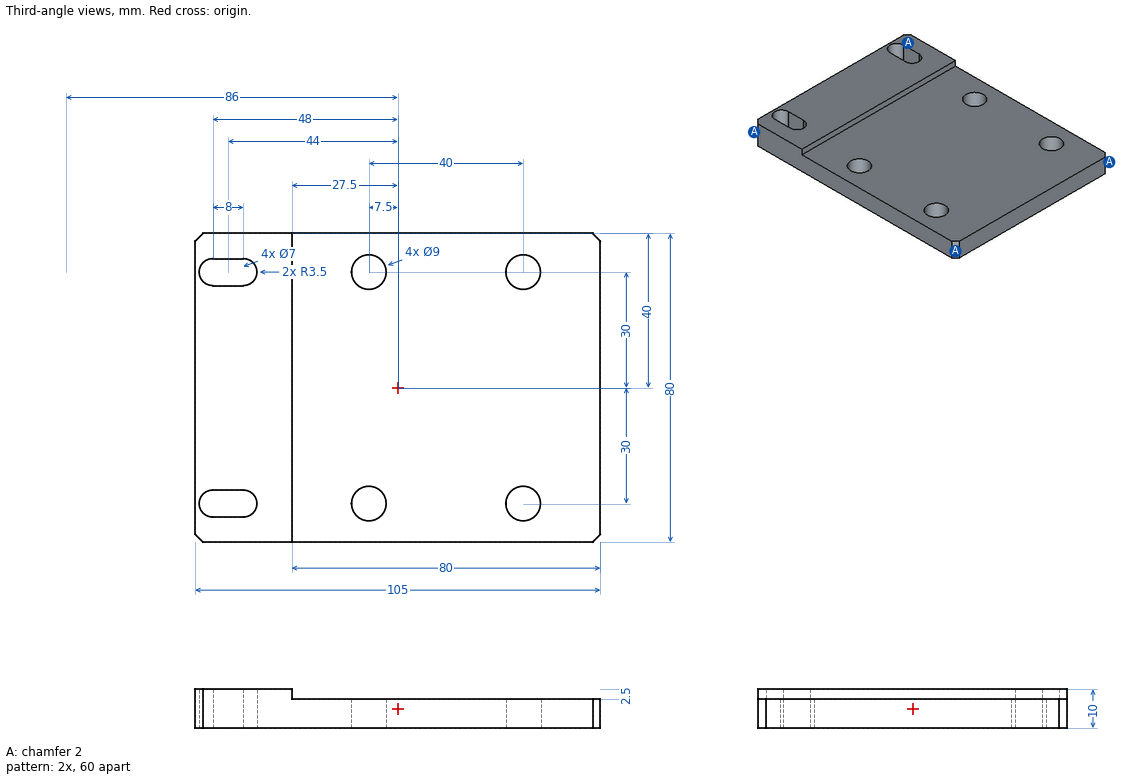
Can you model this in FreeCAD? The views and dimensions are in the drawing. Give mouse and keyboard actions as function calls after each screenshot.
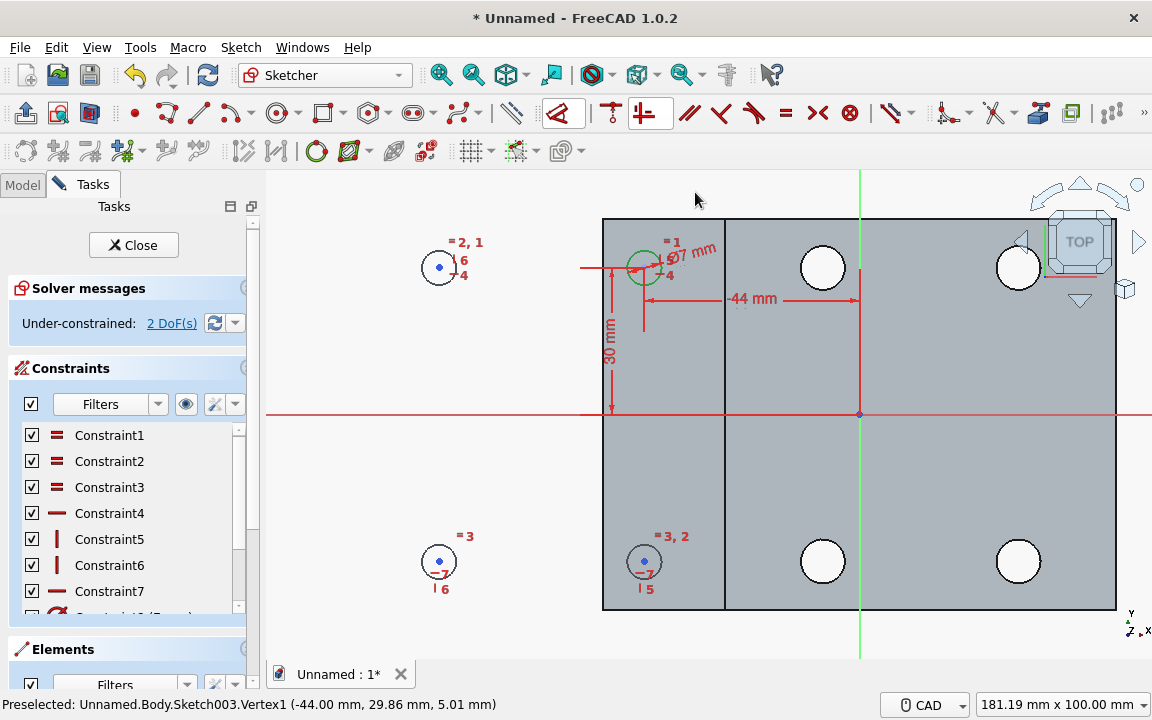
click(439, 268)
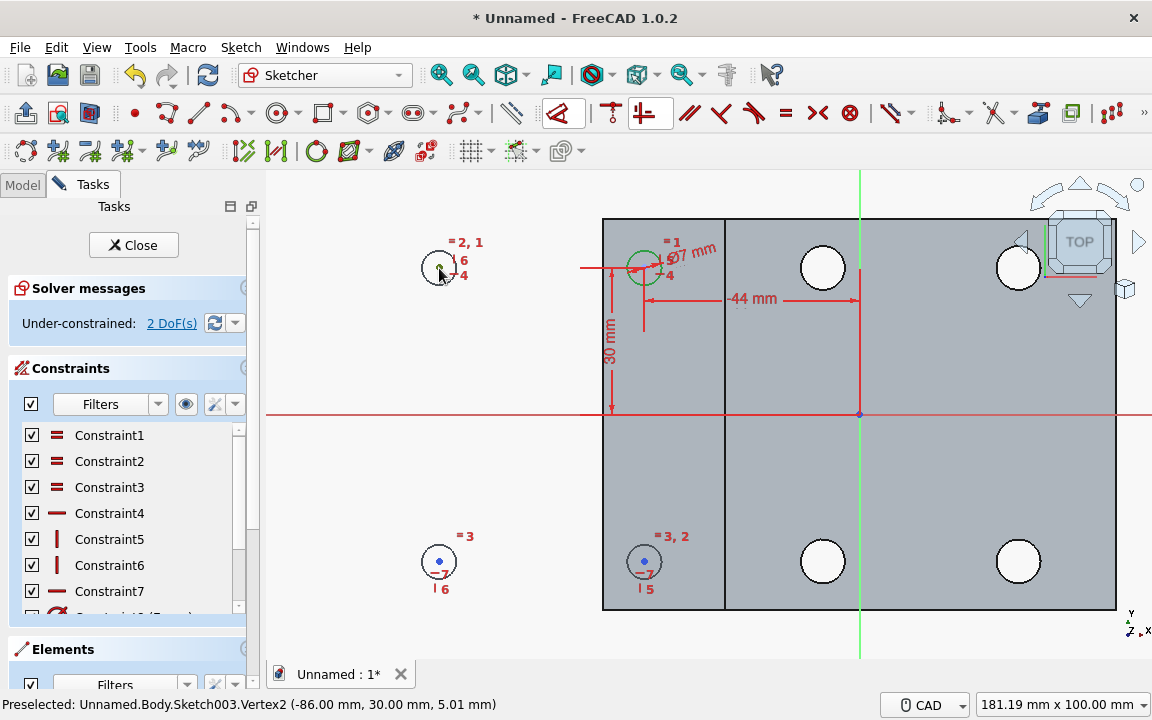
key(l)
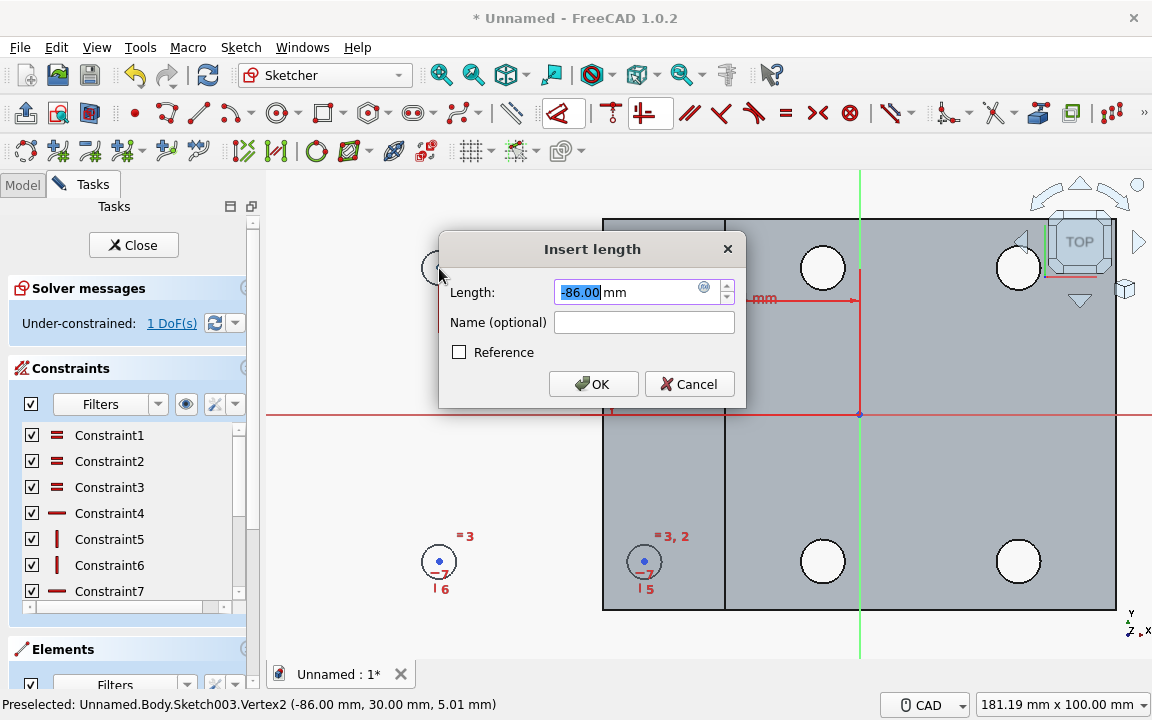
text(-86)
key(Return)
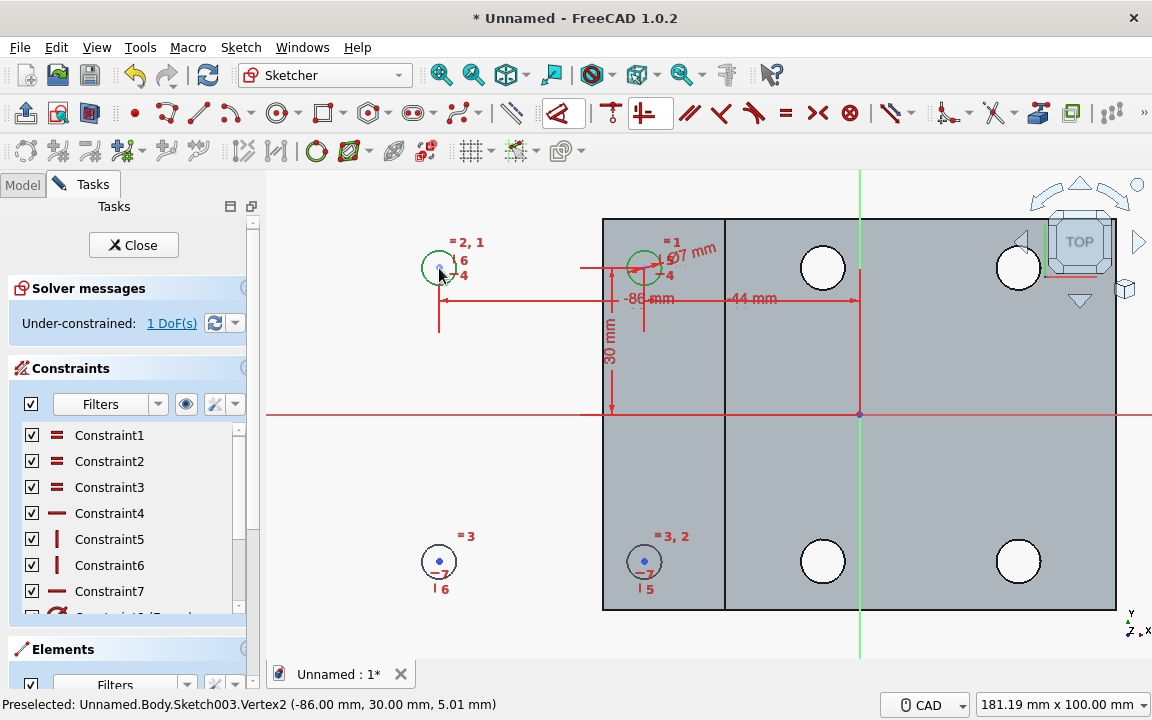
click(644, 562)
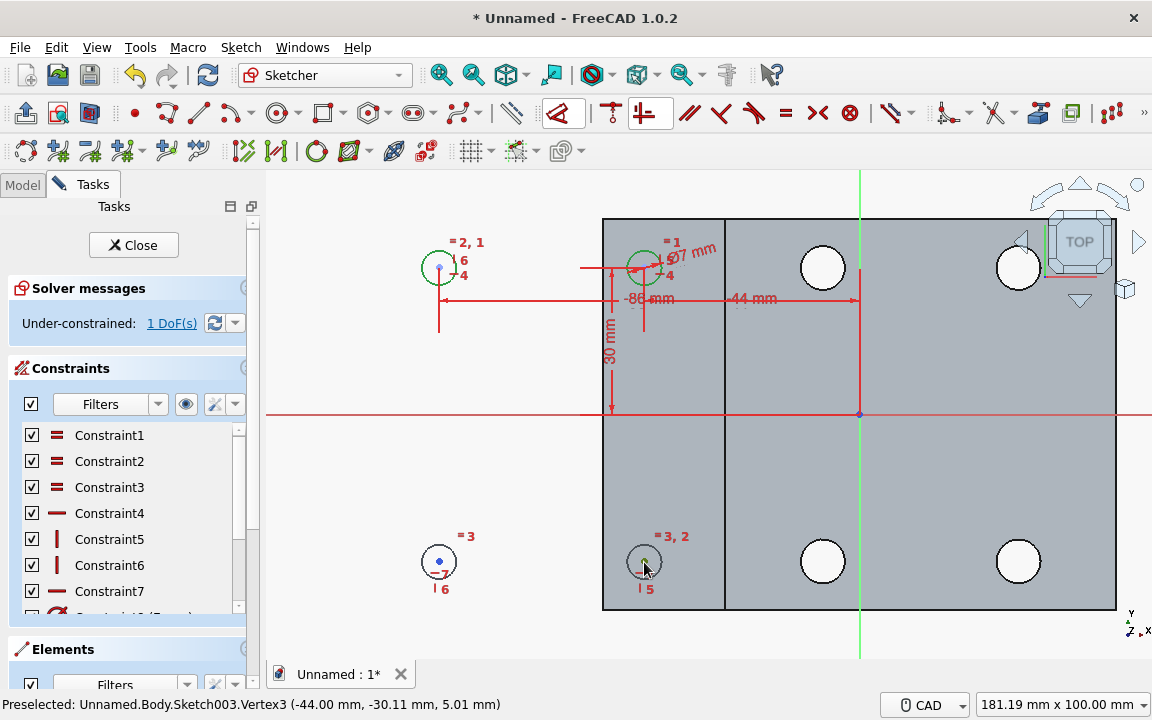
key(i)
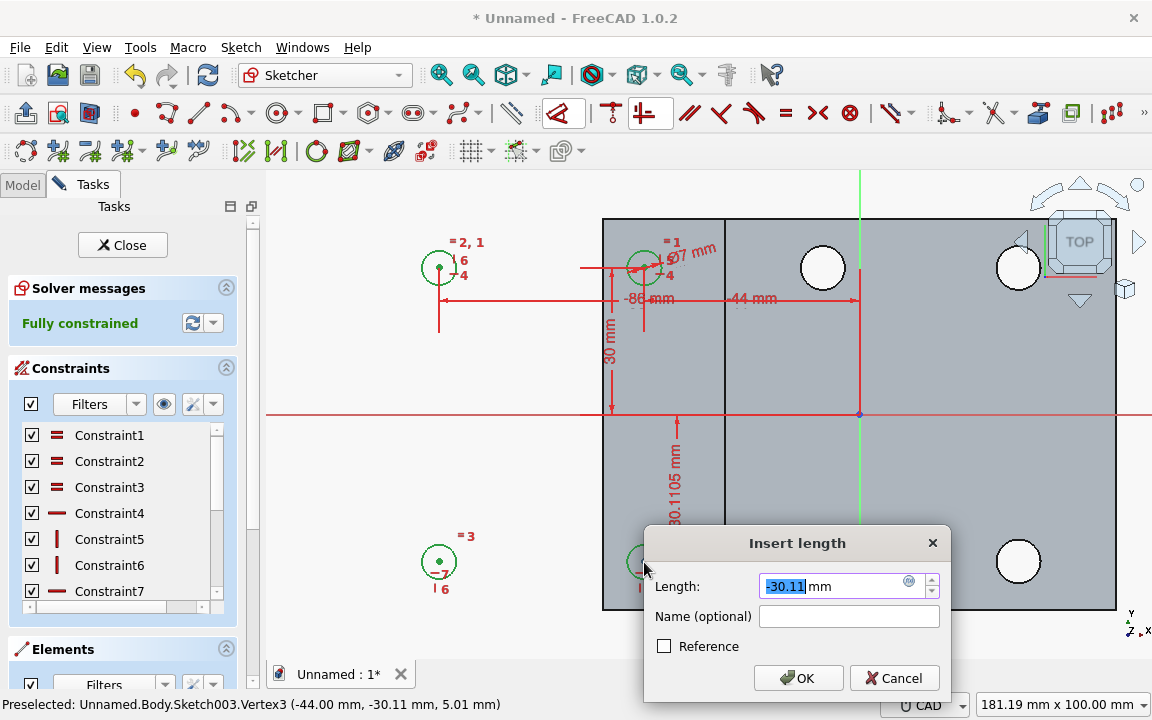
text(-30)
key(Return)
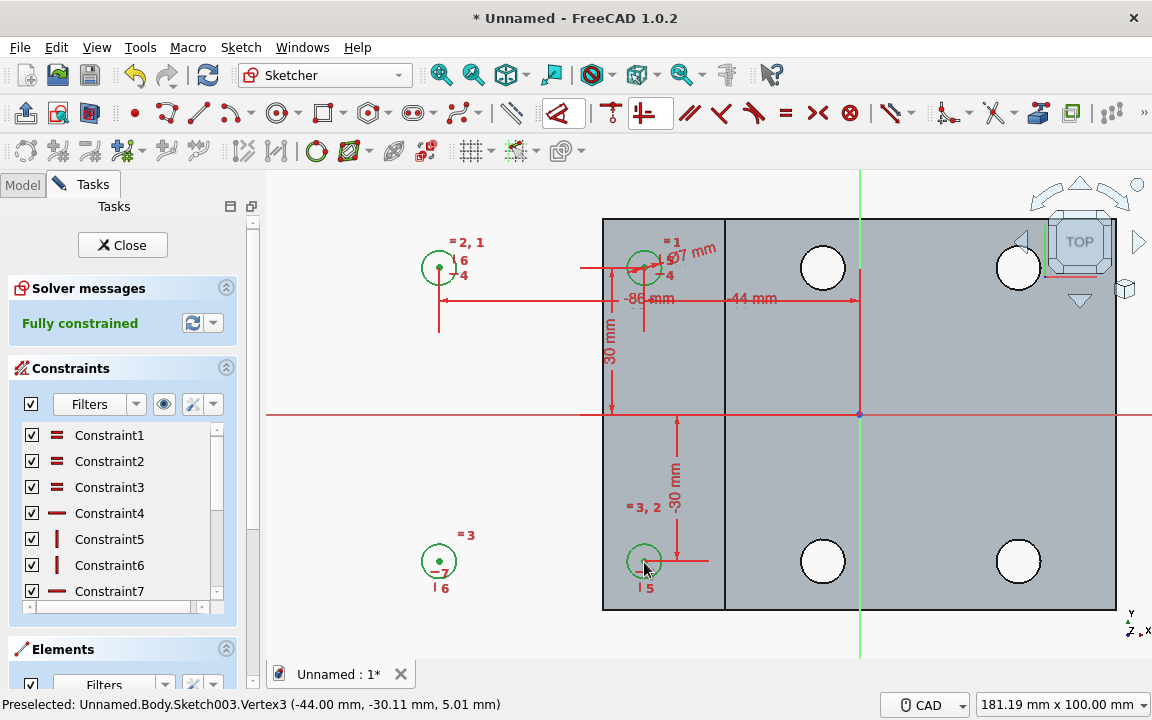
click(123, 245)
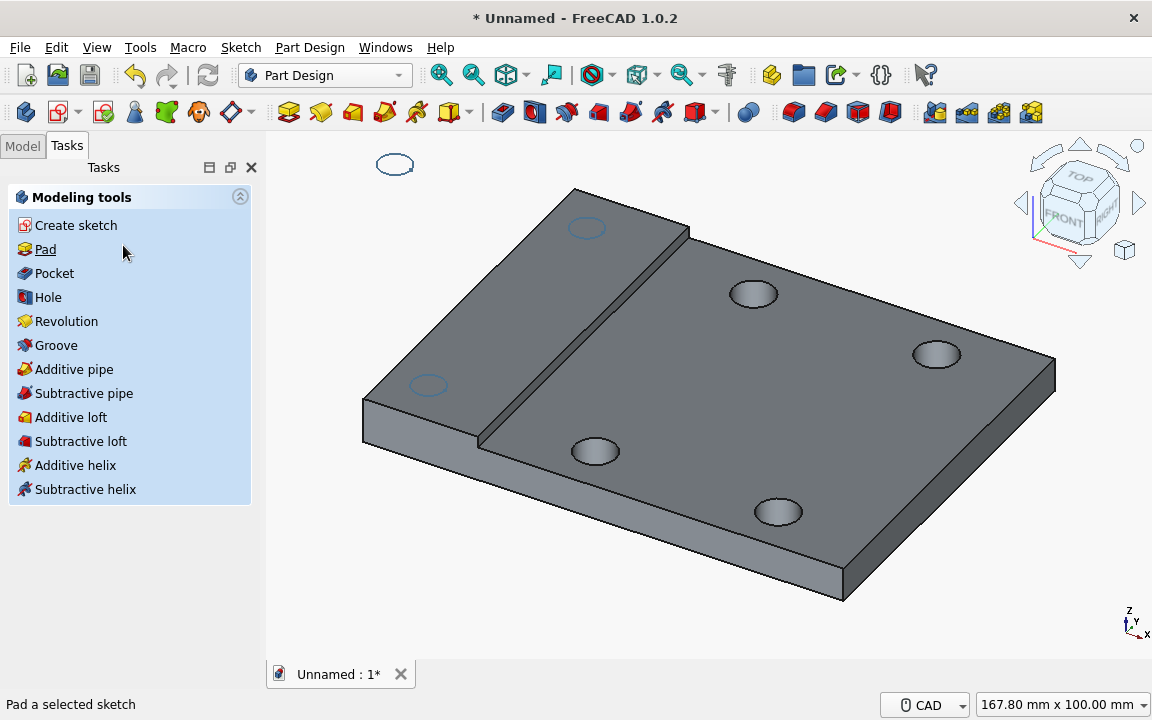
click(504, 112)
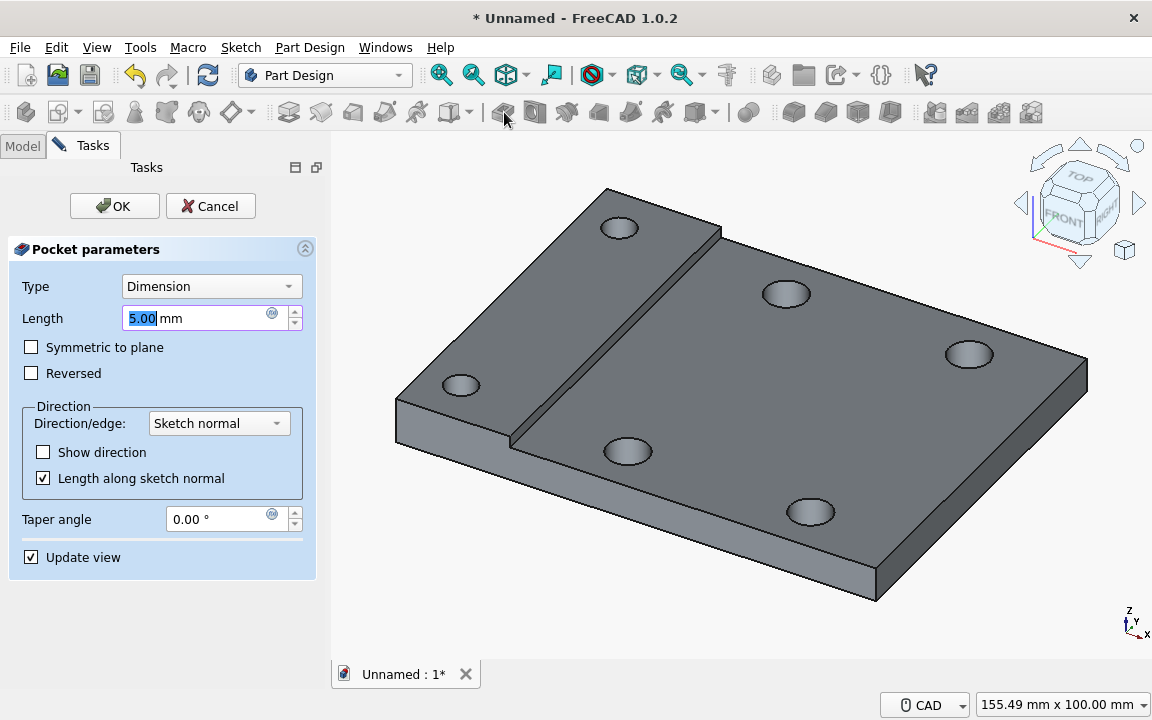
click(212, 286)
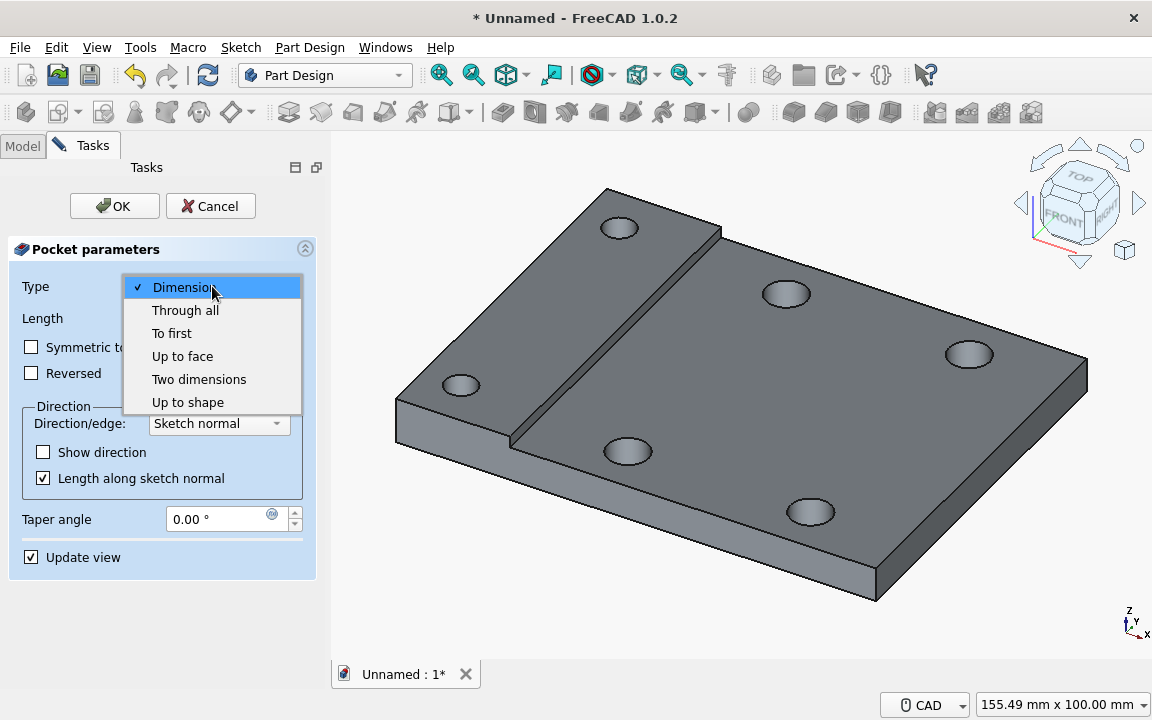
click(212, 310)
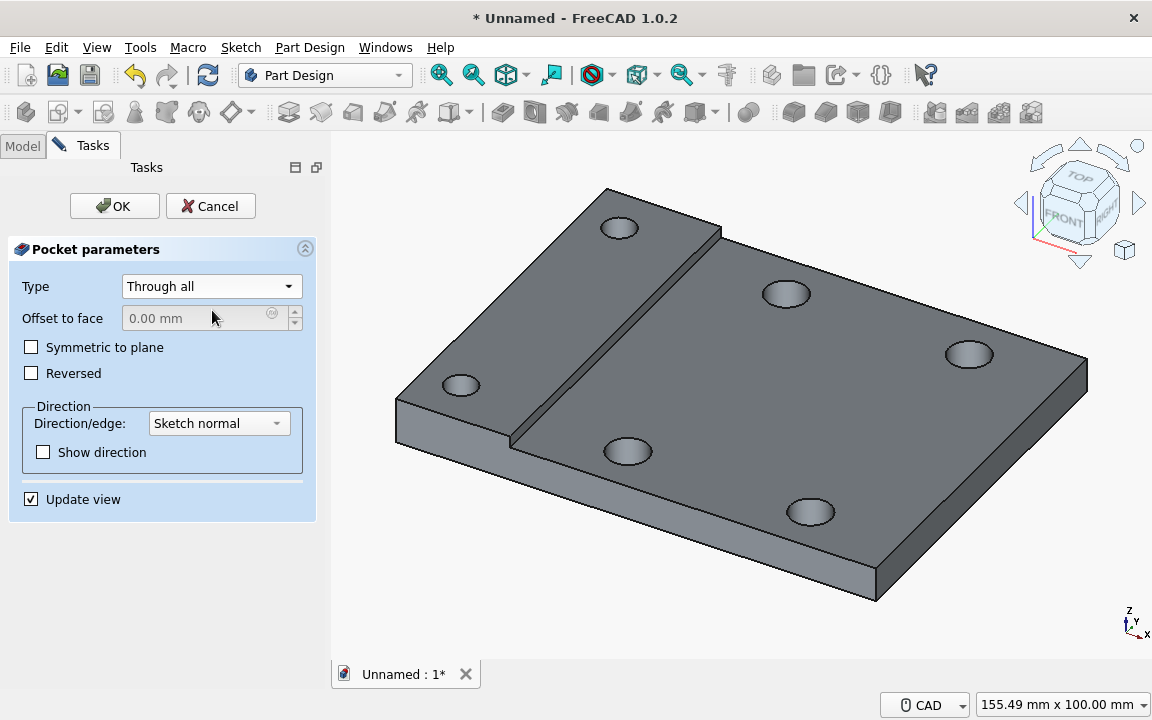
click(115, 206)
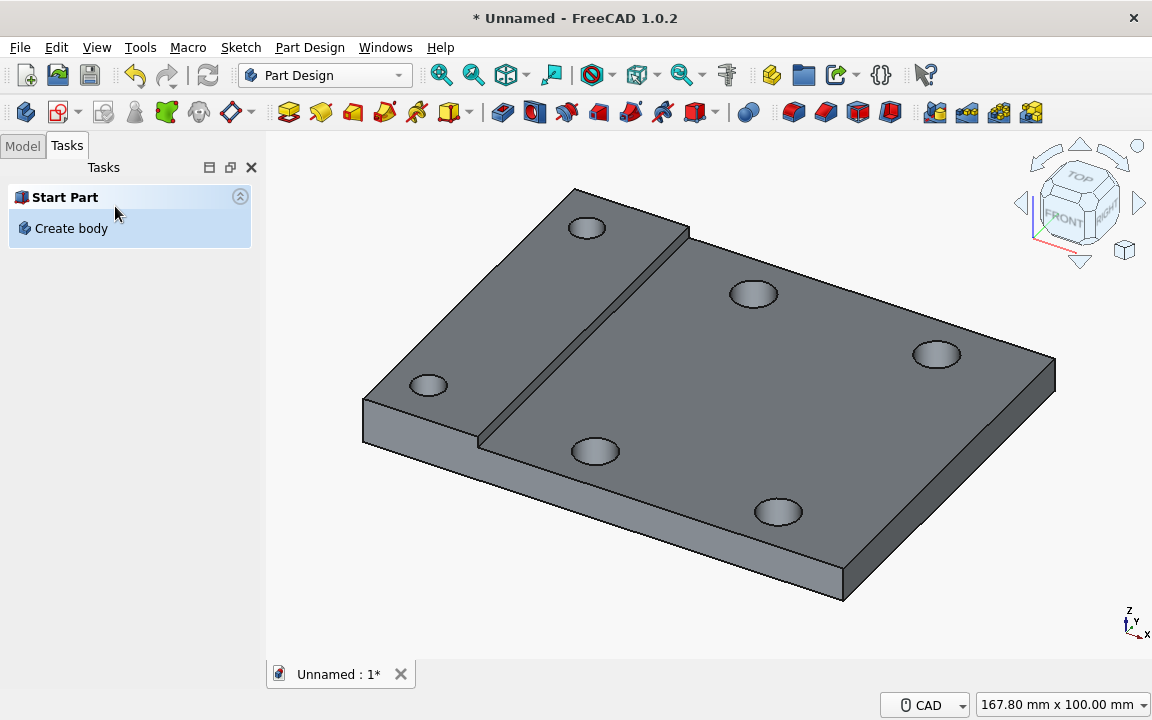
click(843, 584)